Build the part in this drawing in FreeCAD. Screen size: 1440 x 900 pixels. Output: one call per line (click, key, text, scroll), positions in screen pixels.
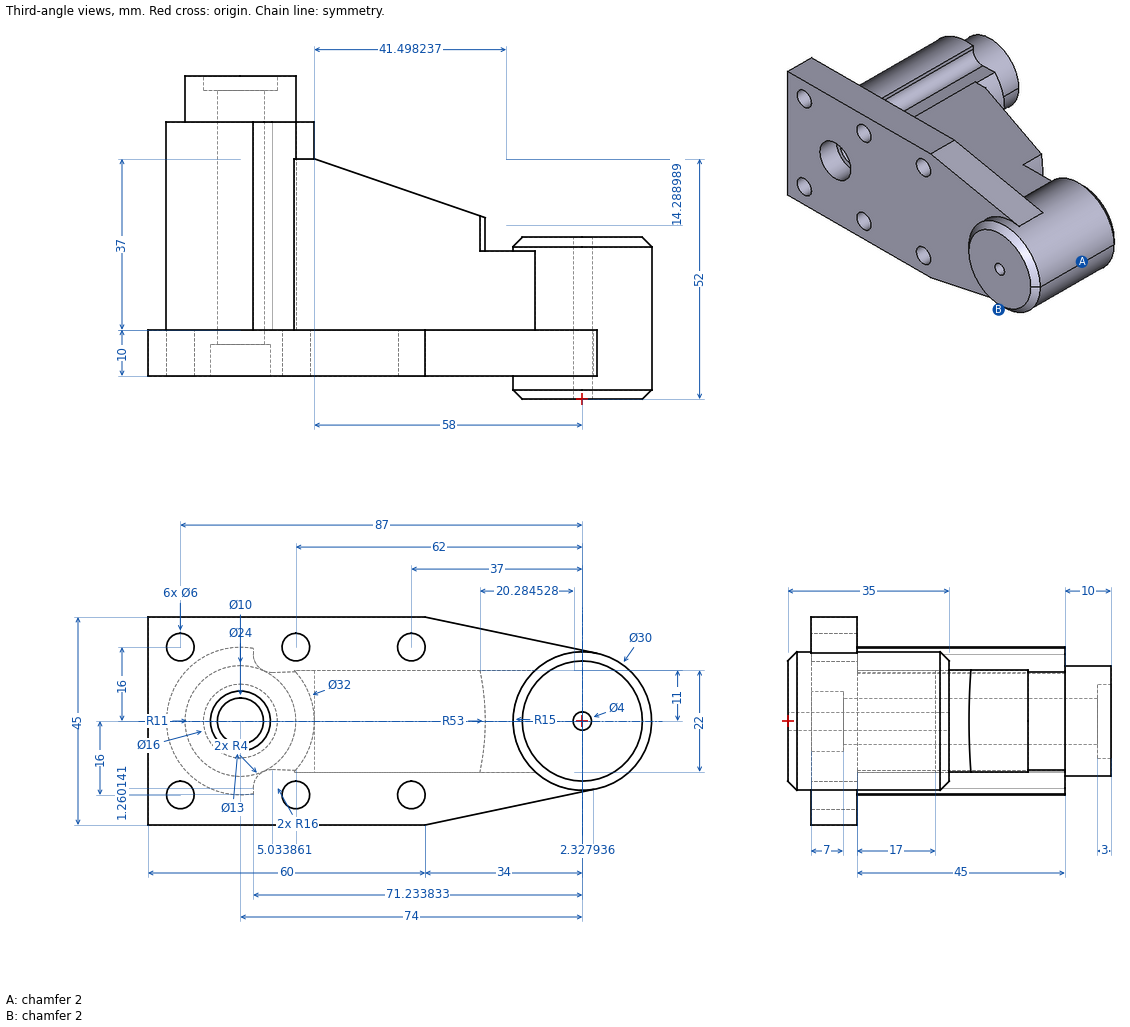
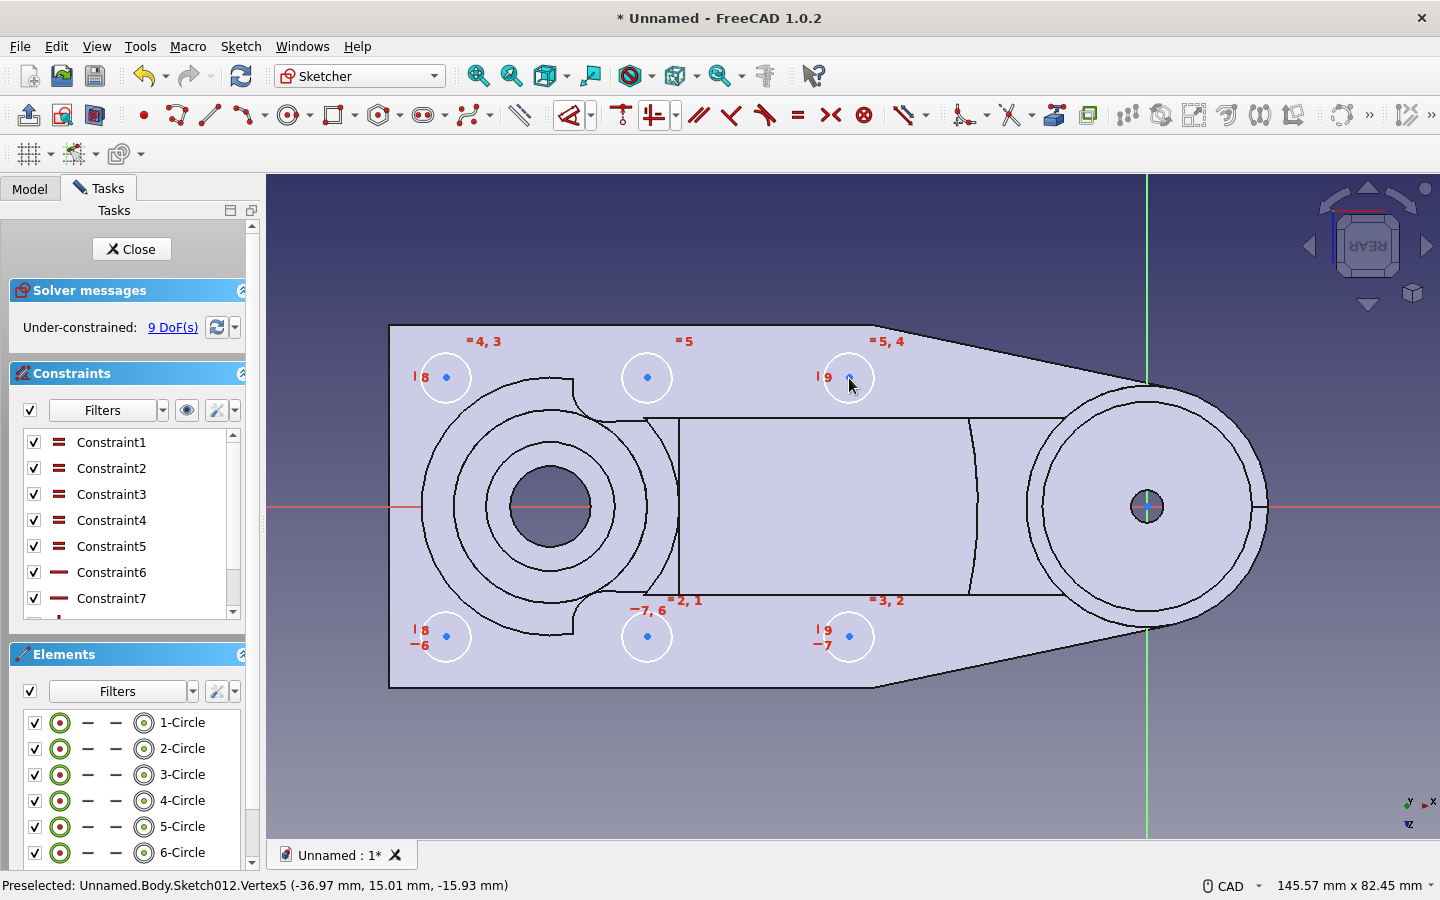
click(446, 378)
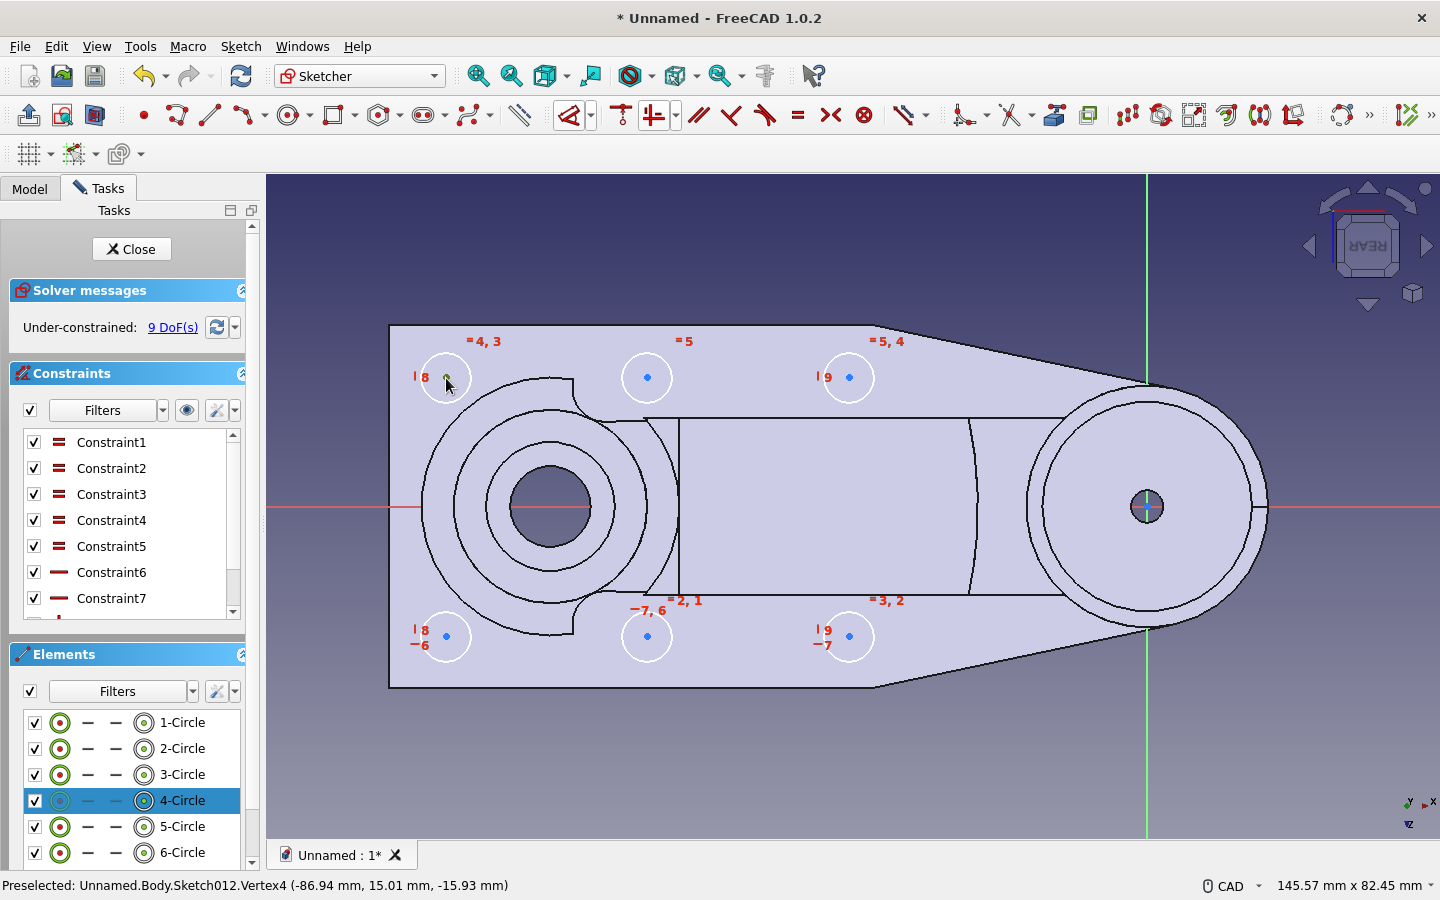
click(849, 378)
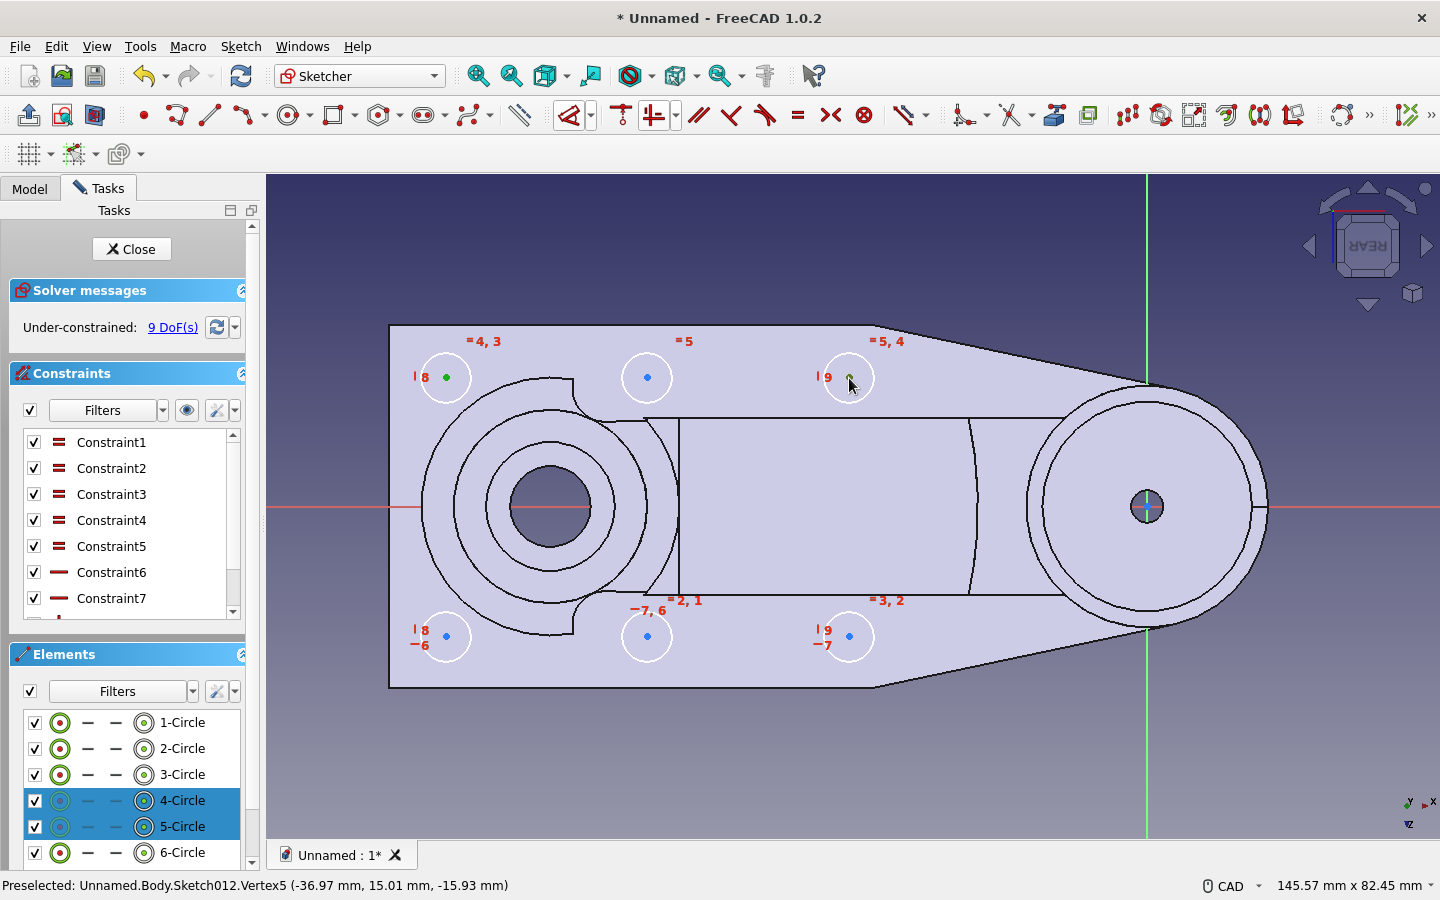
key(h)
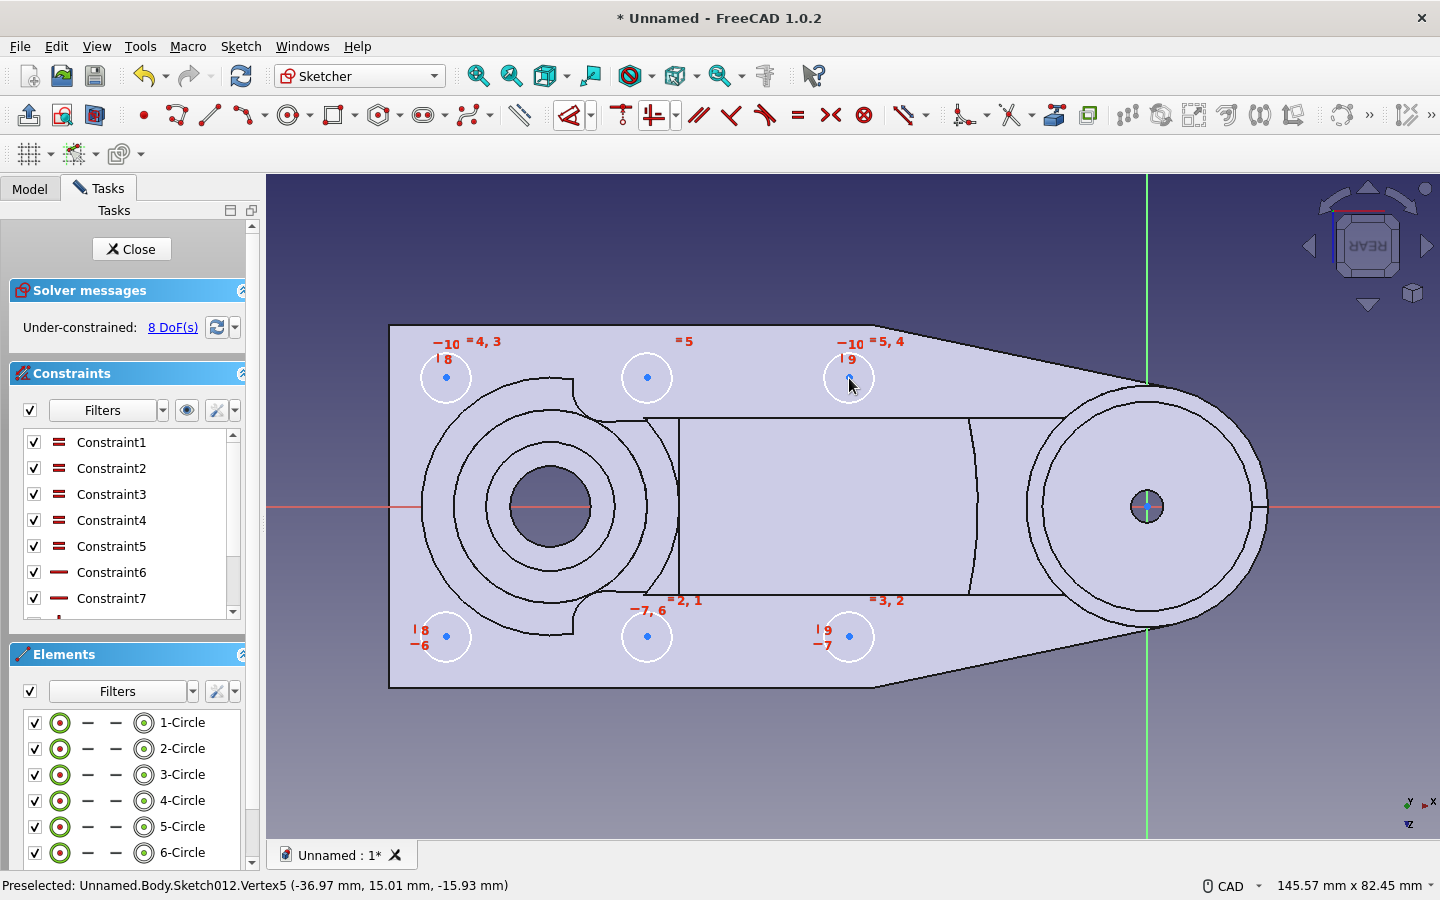
click(647, 637)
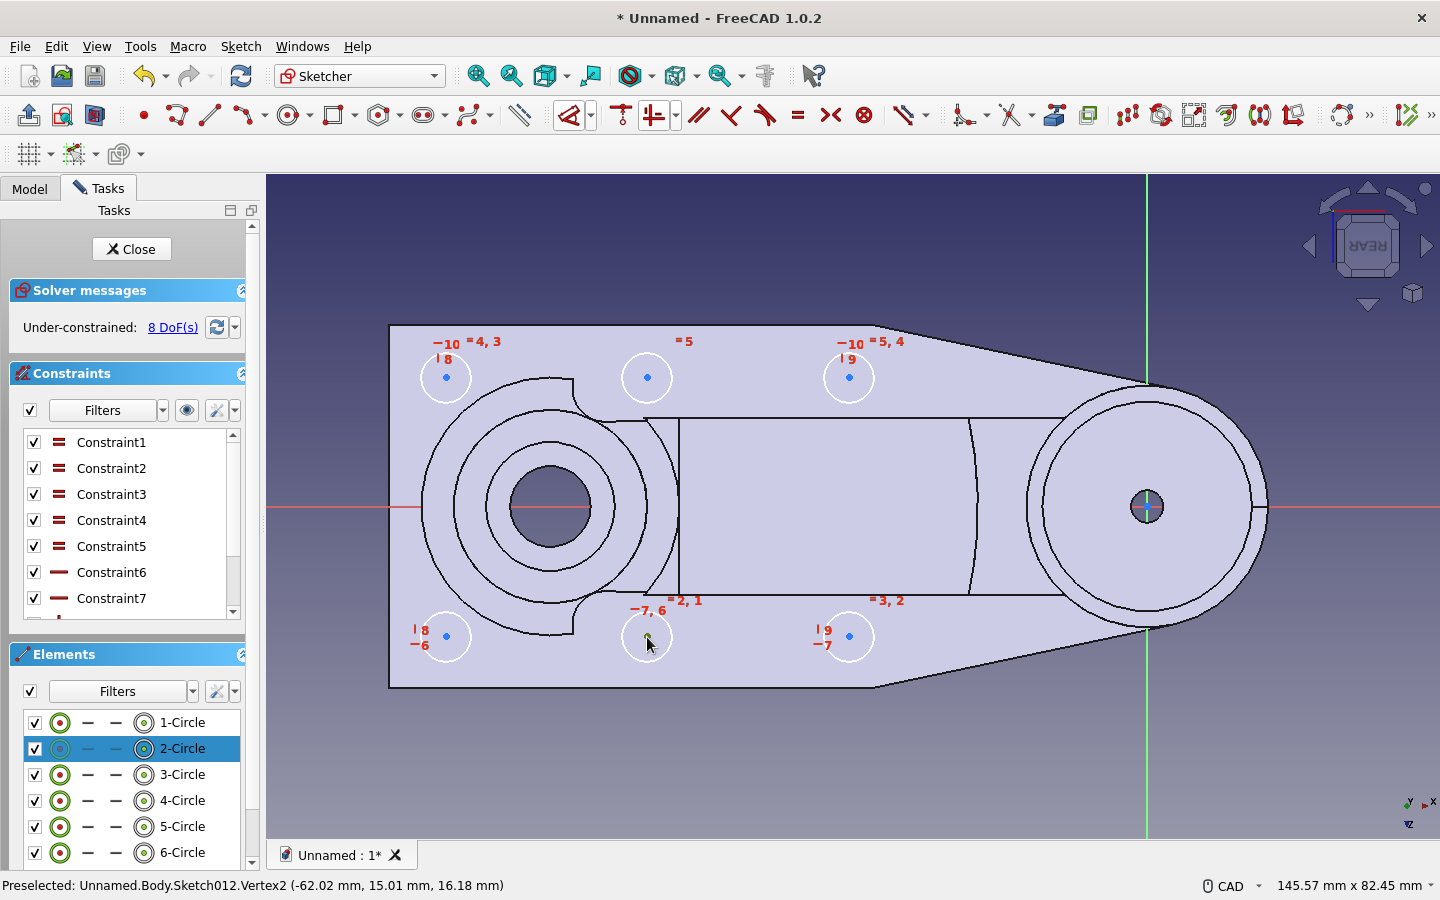
click(647, 378)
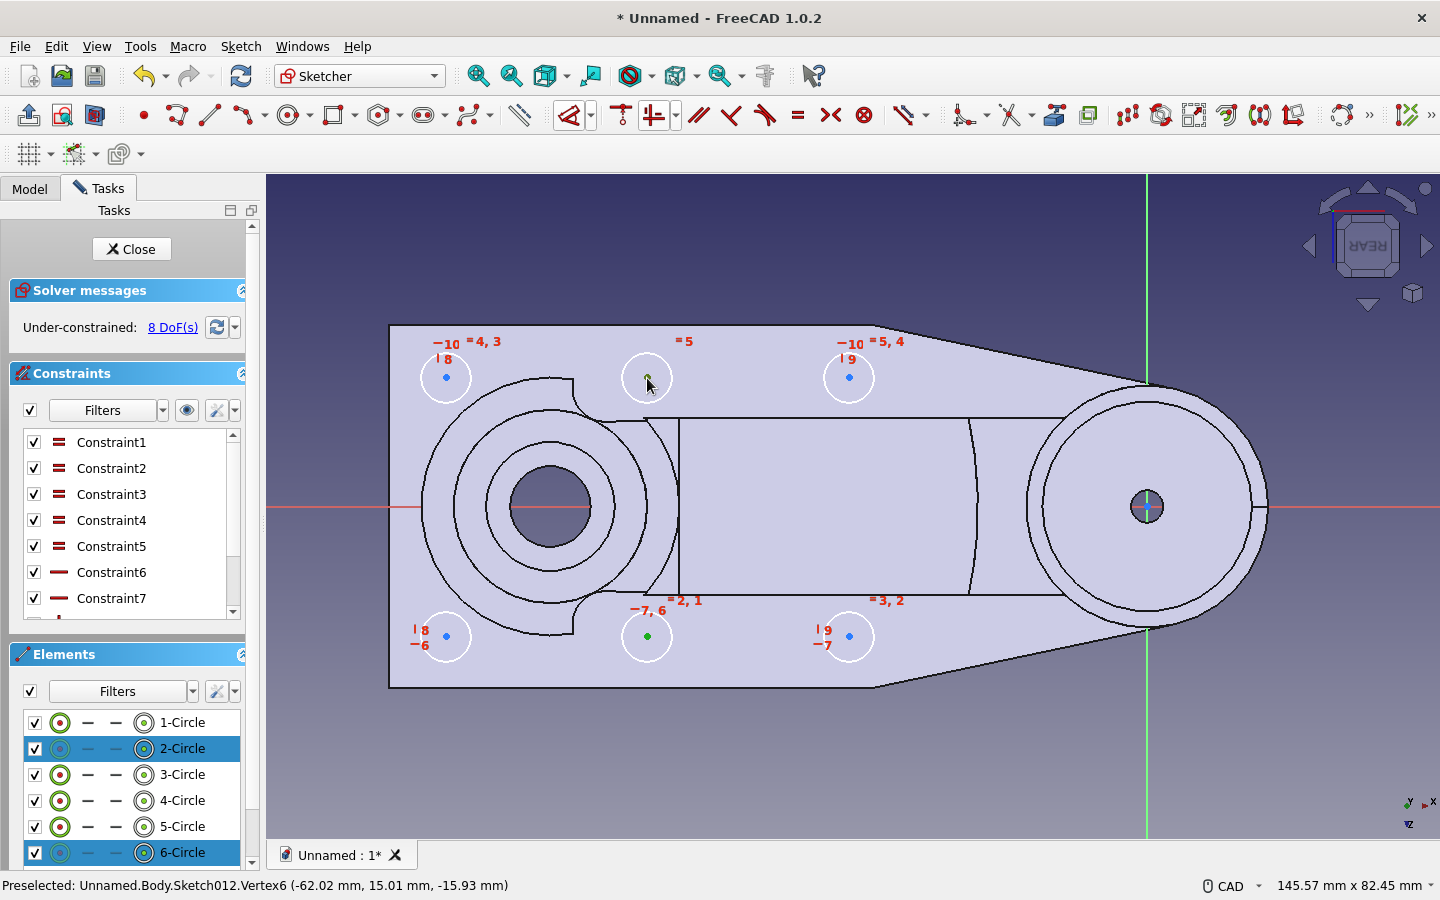
key(v)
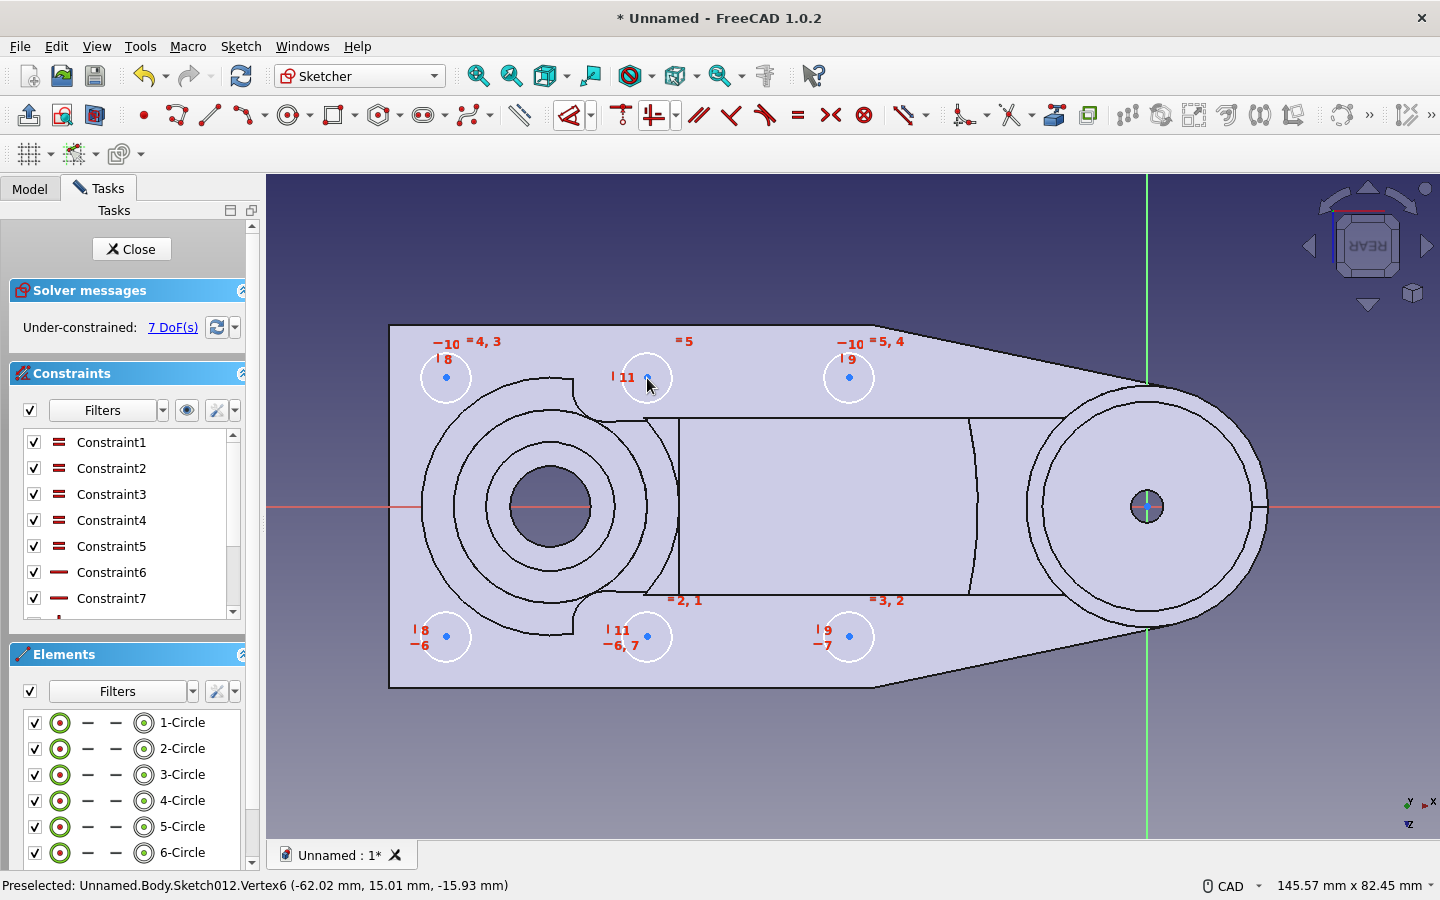
click(446, 378)